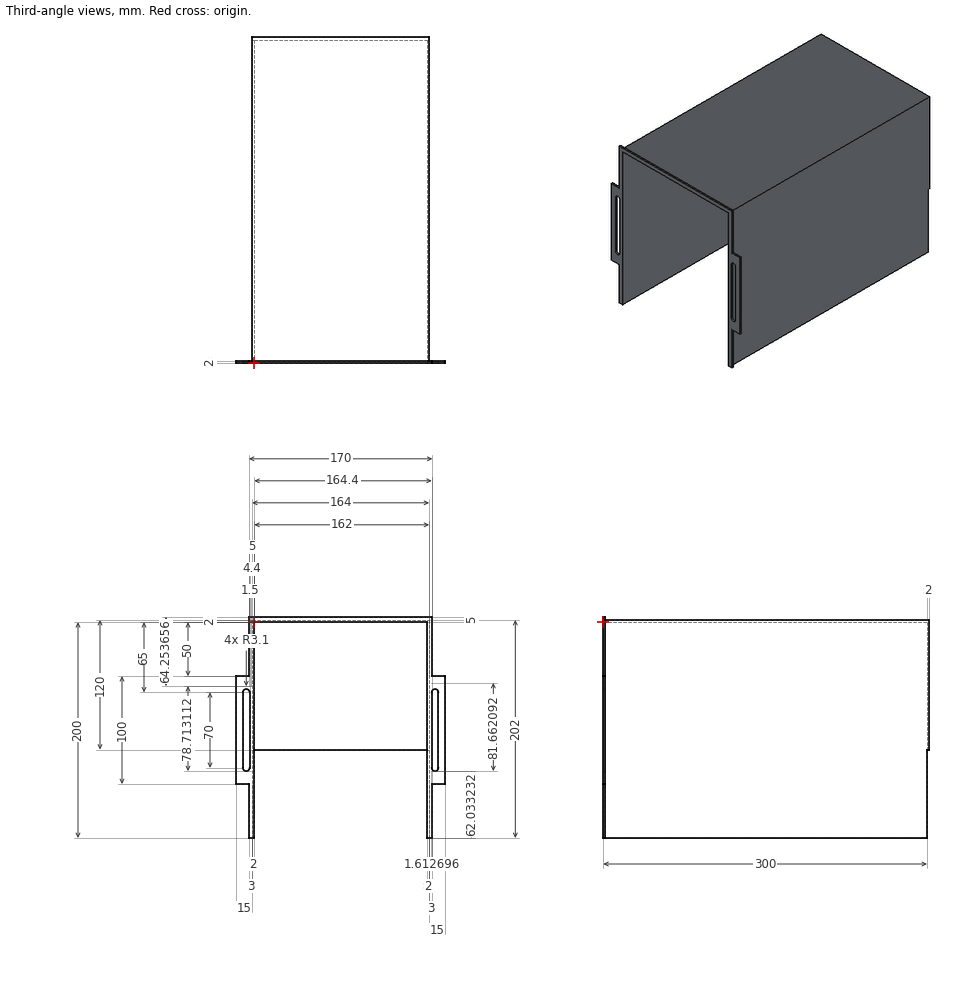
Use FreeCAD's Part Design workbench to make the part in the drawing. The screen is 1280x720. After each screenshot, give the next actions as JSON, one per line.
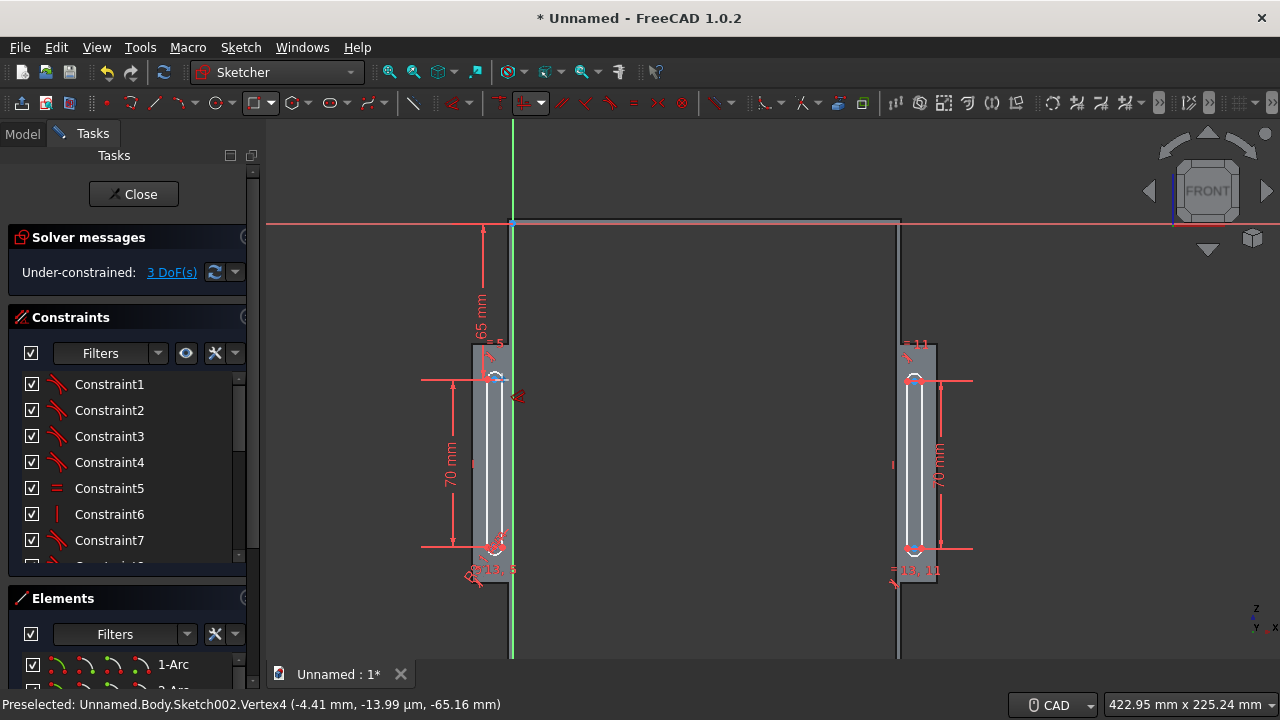
{"action": "scroll", "coordinate": [922, 381], "scroll_direction": "up", "scroll_amount": 3}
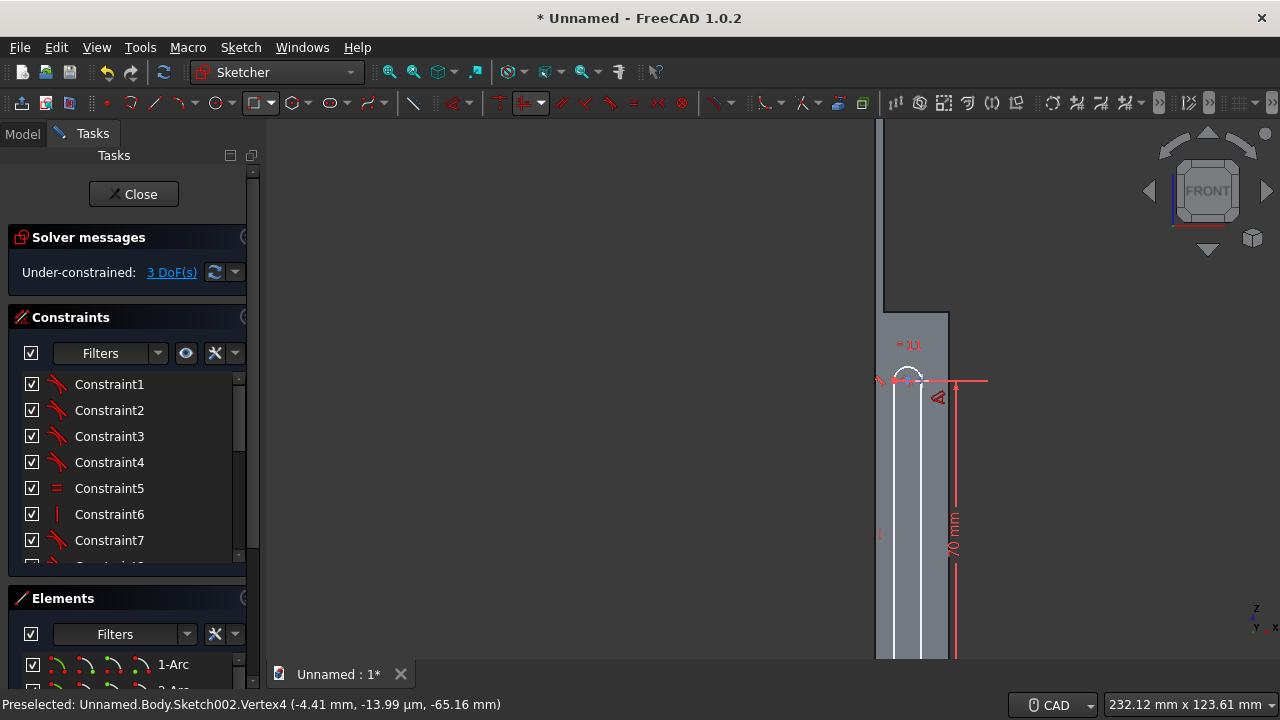
{"action": "left_click", "coordinate": [921, 381]}
{"action": "left_click", "coordinate": [955, 264]}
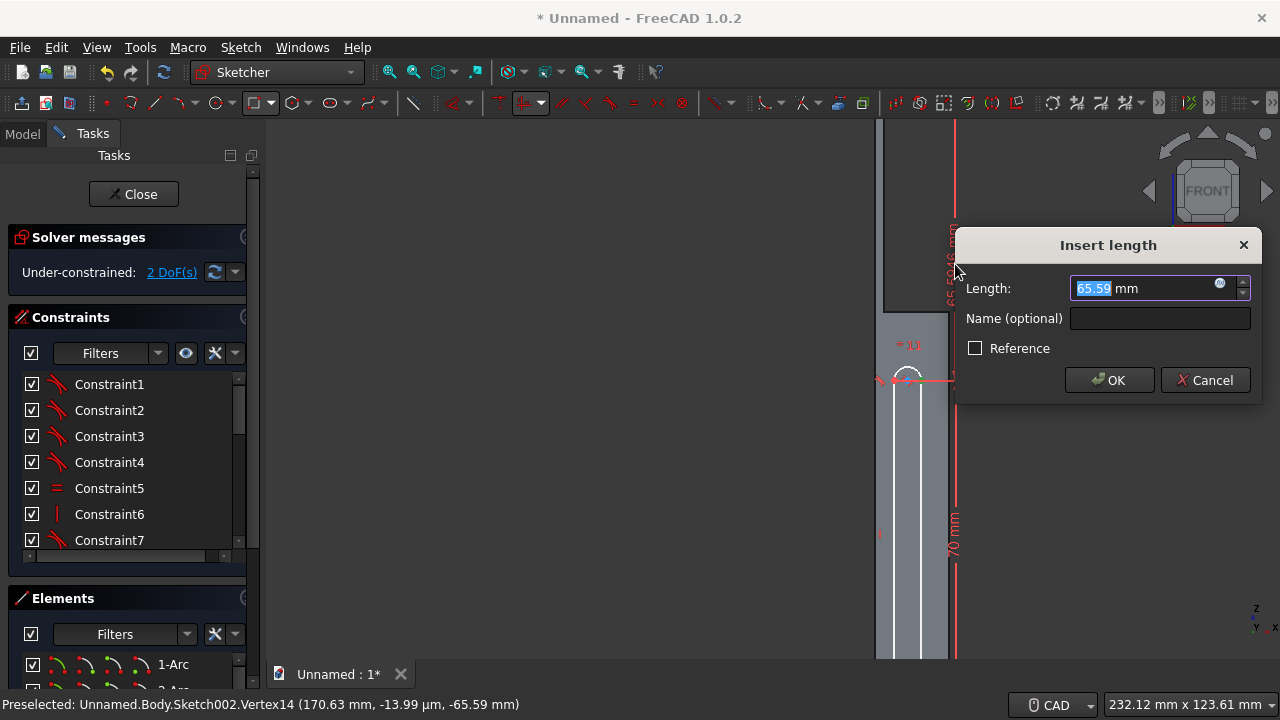
{"action": "type", "text": "65"}
{"action": "key", "text": "Return"}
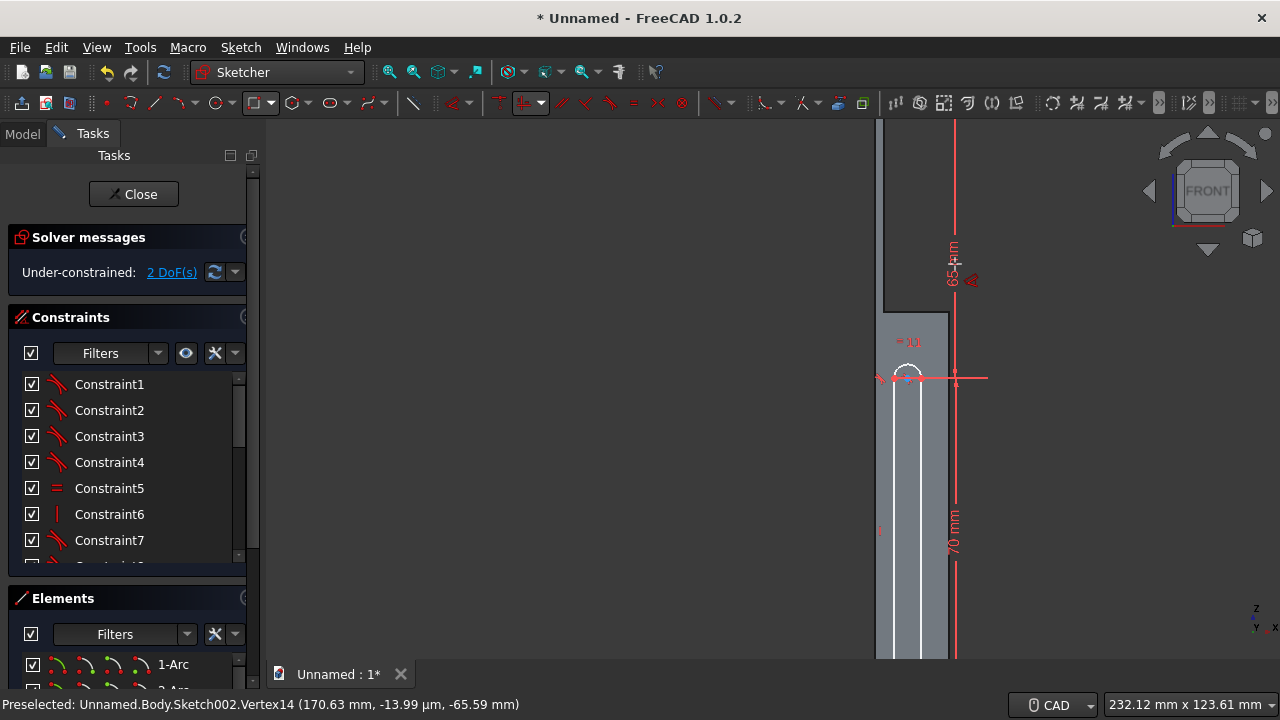
{"action": "scroll", "coordinate": [922, 381], "scroll_direction": "down", "scroll_amount": 3}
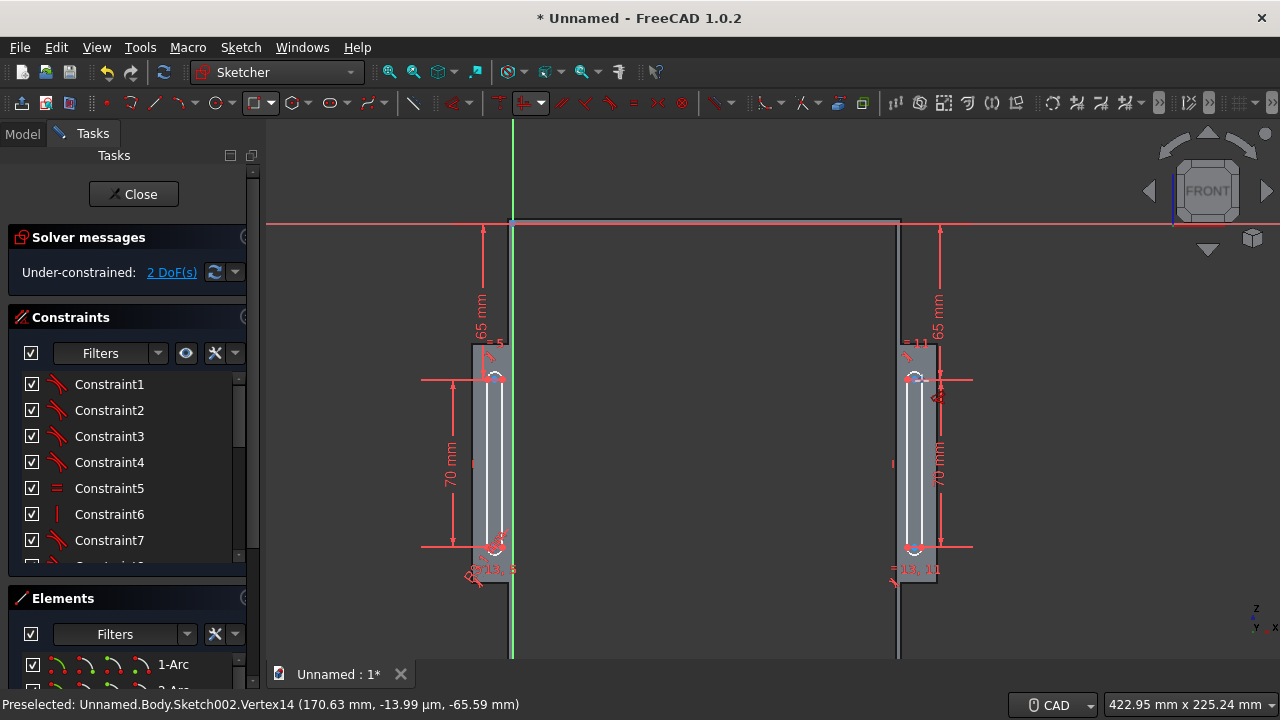
{"action": "scroll", "coordinate": [502, 547], "scroll_direction": "up", "scroll_amount": 7}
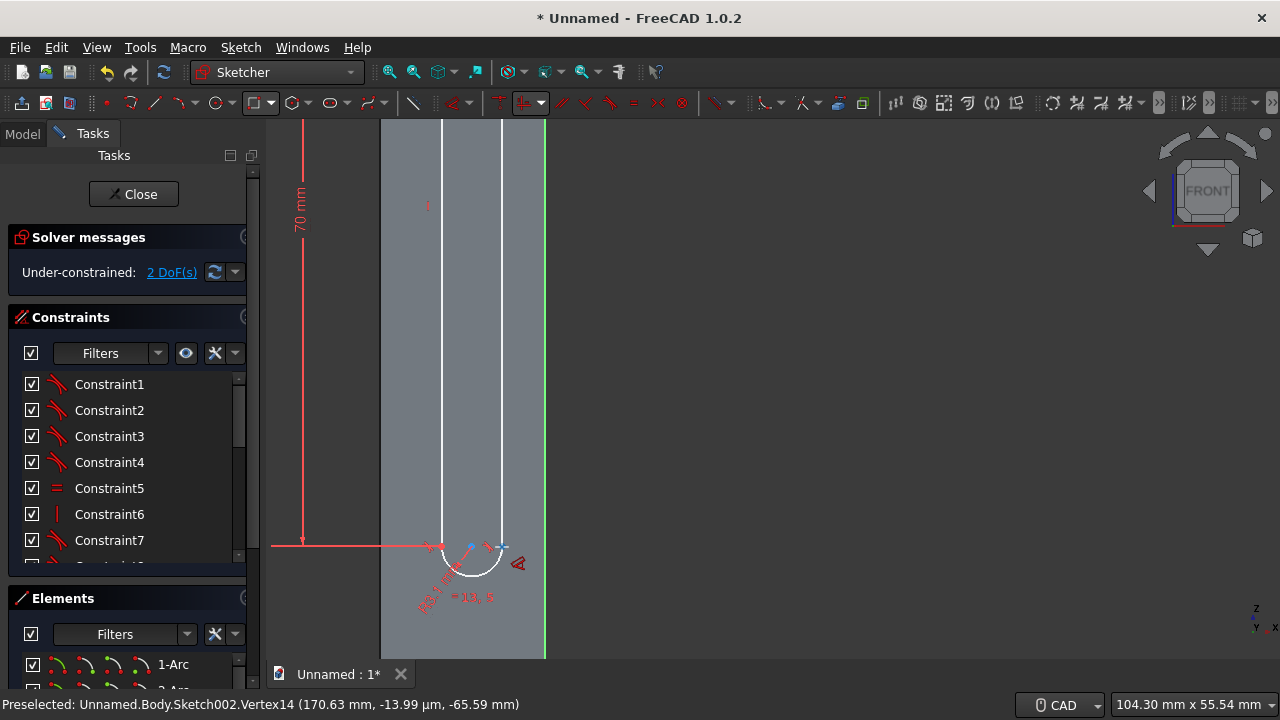
{"action": "left_click", "coordinate": [502, 546]}
{"action": "left_click", "coordinate": [524, 580]}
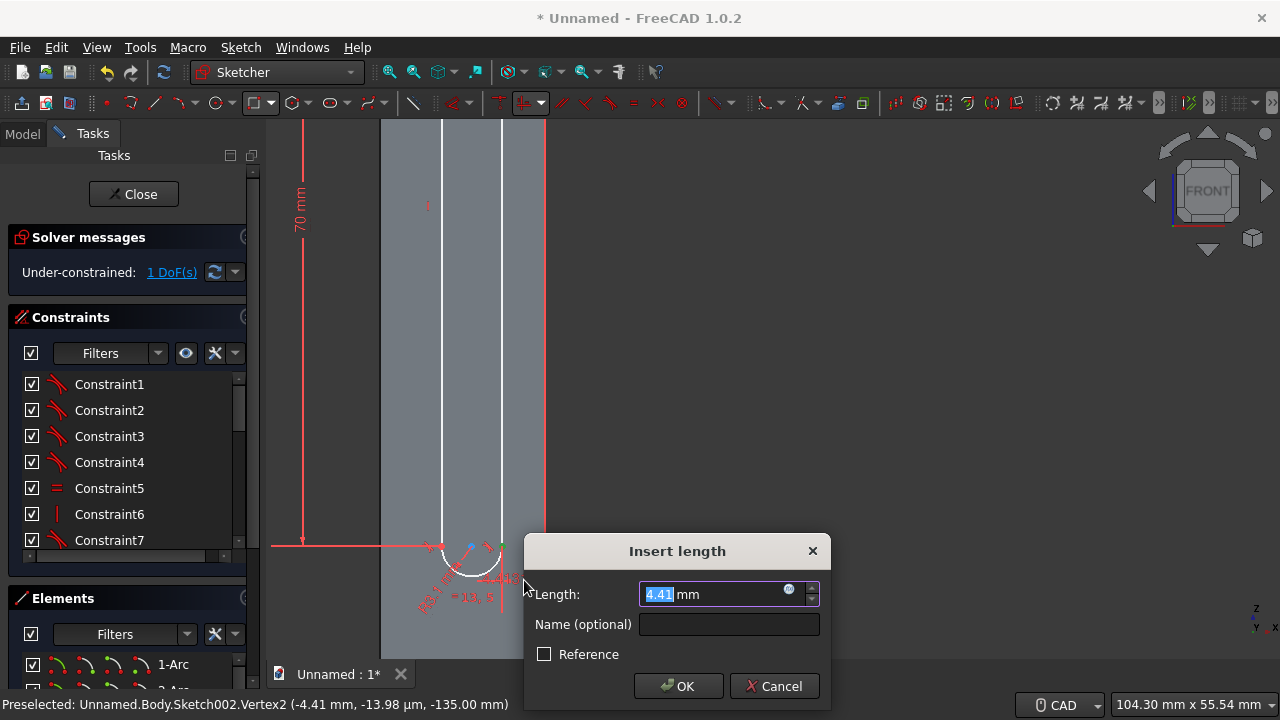
{"action": "type", "text": "4.4"}
{"action": "key", "text": "Return"}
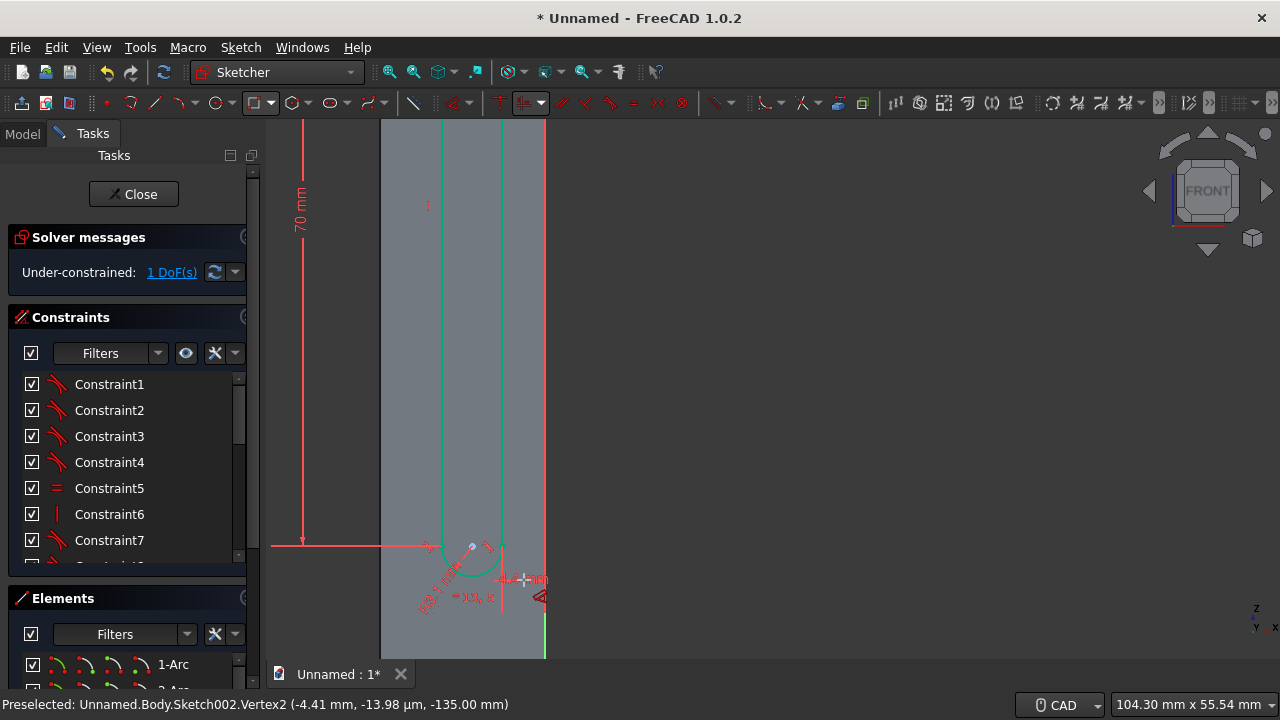
{"action": "scroll", "coordinate": [502, 547], "scroll_direction": "down", "scroll_amount": 7}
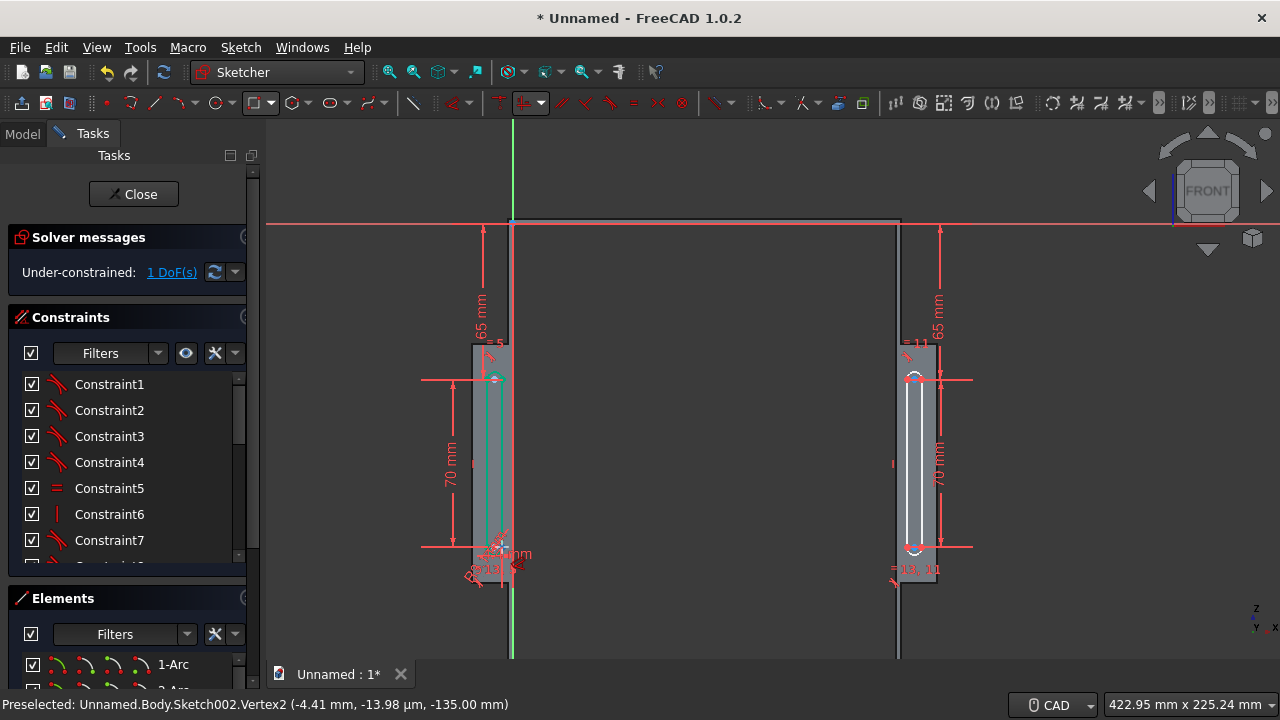
{"action": "scroll", "coordinate": [907, 547], "scroll_direction": "up", "scroll_amount": 3}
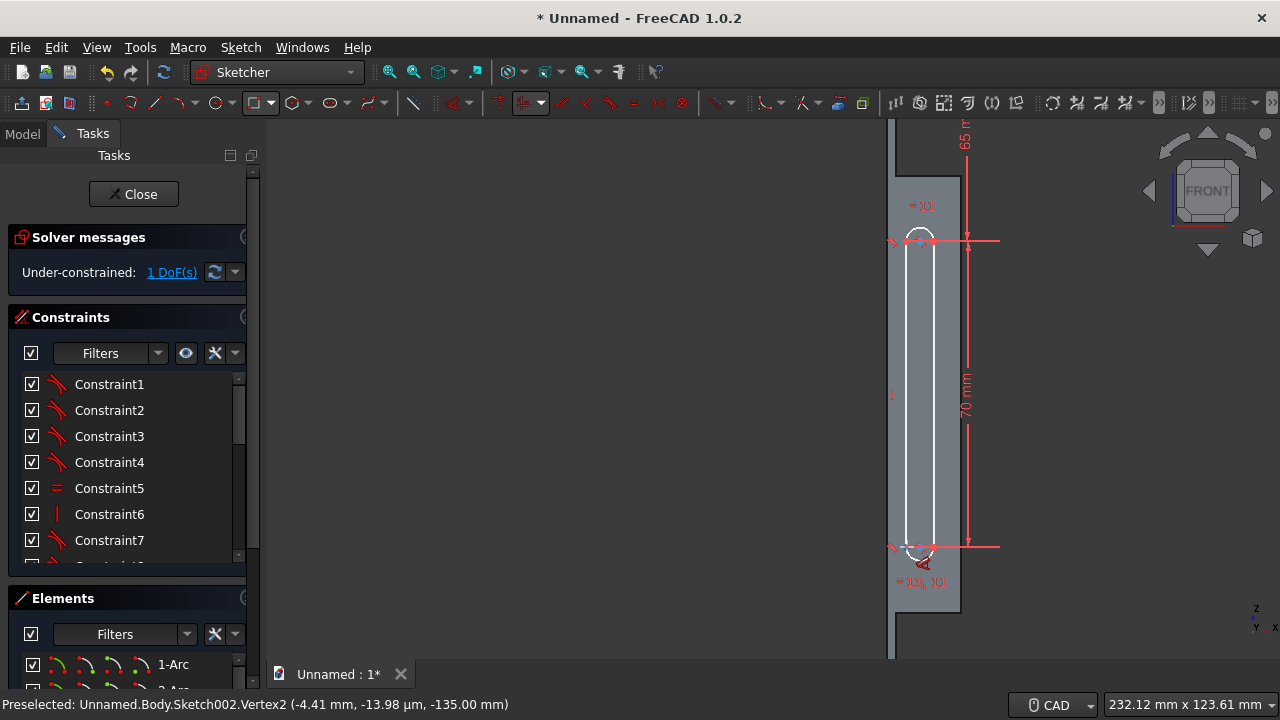
{"action": "left_click", "coordinate": [906, 547]}
{"action": "left_click", "coordinate": [600, 581]}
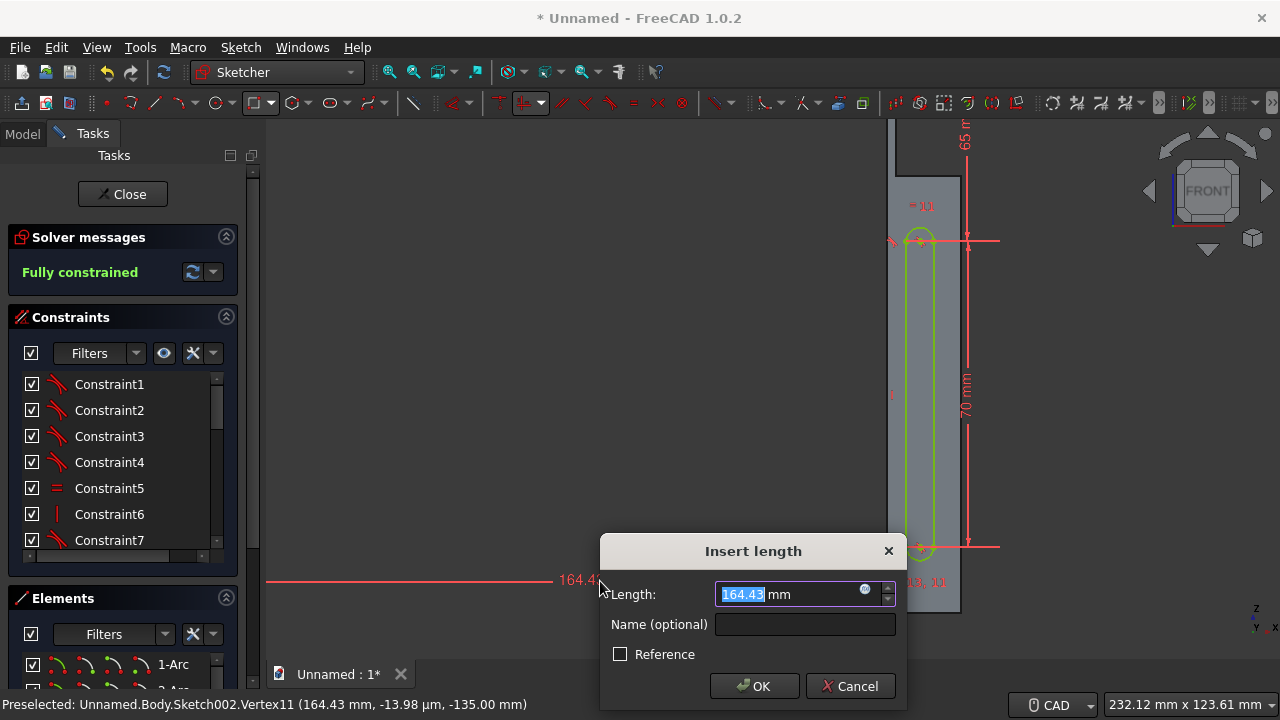
{"action": "type", "text": "164.4"}
{"action": "key", "text": "Return"}
{"action": "key", "text": "Escape"}